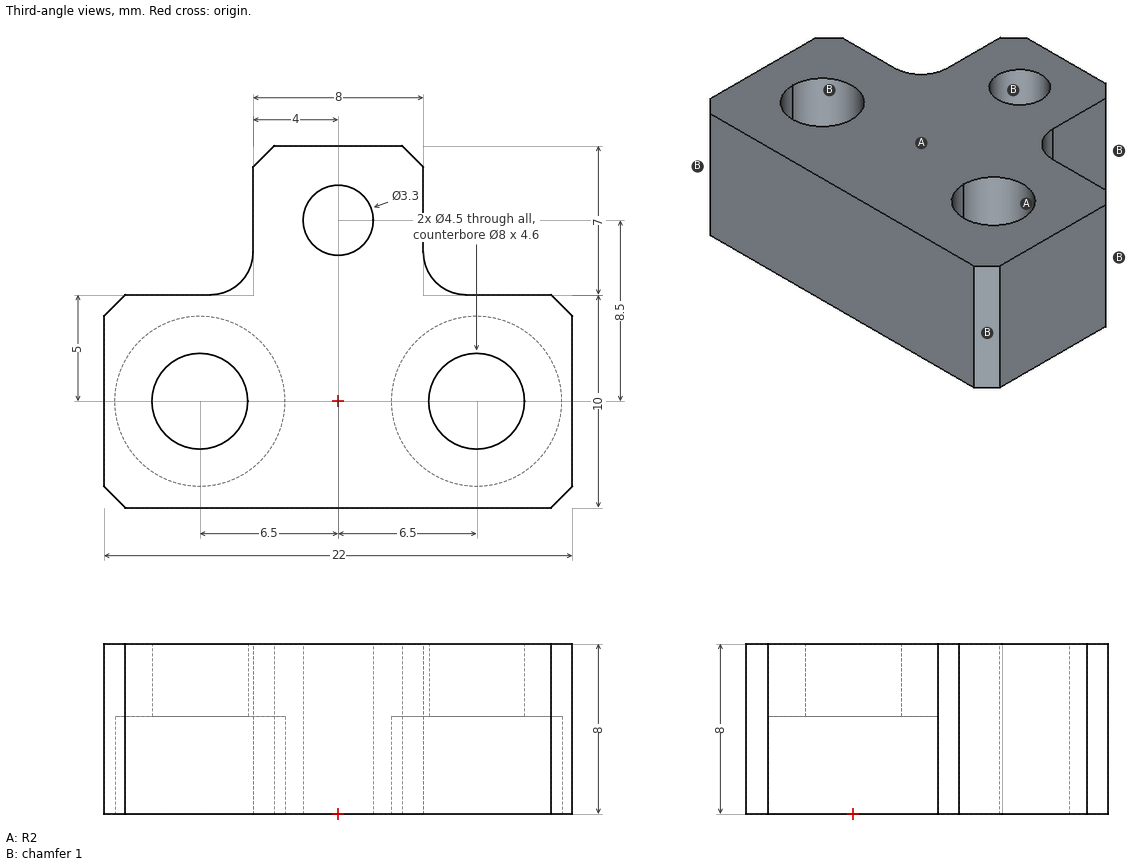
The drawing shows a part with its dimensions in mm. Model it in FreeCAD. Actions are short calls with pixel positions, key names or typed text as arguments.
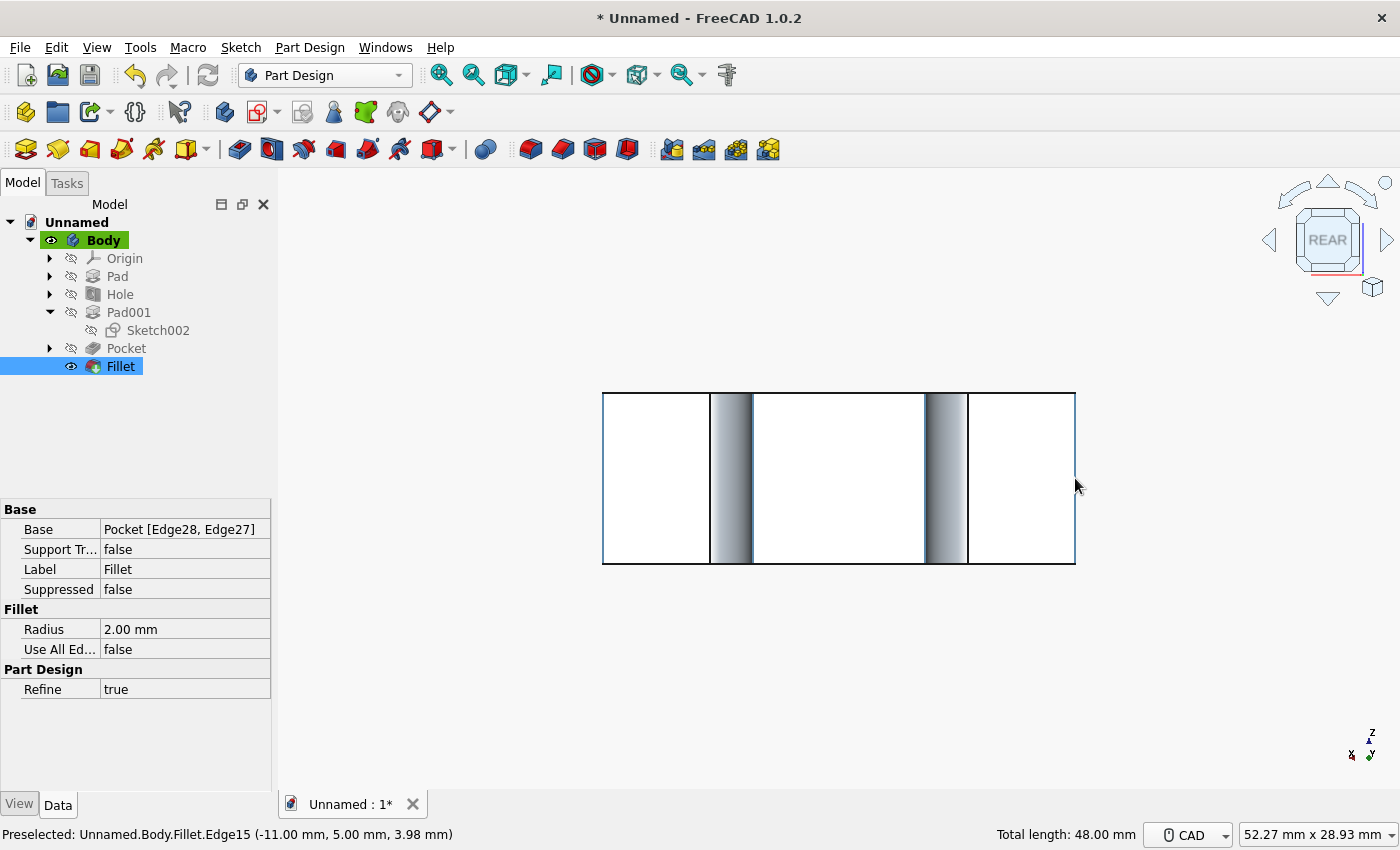
click(564, 150)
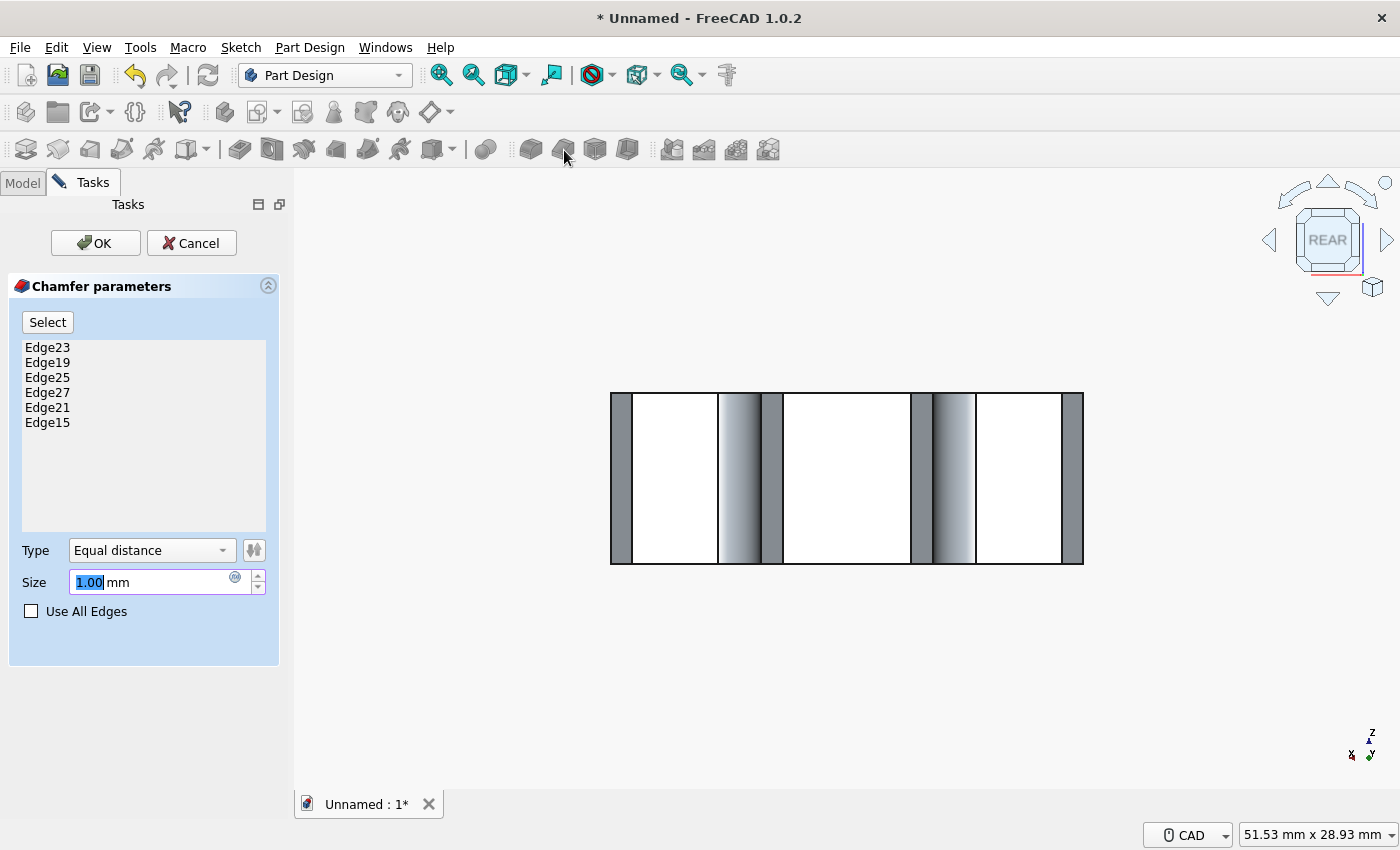
text(1)
key(Tab)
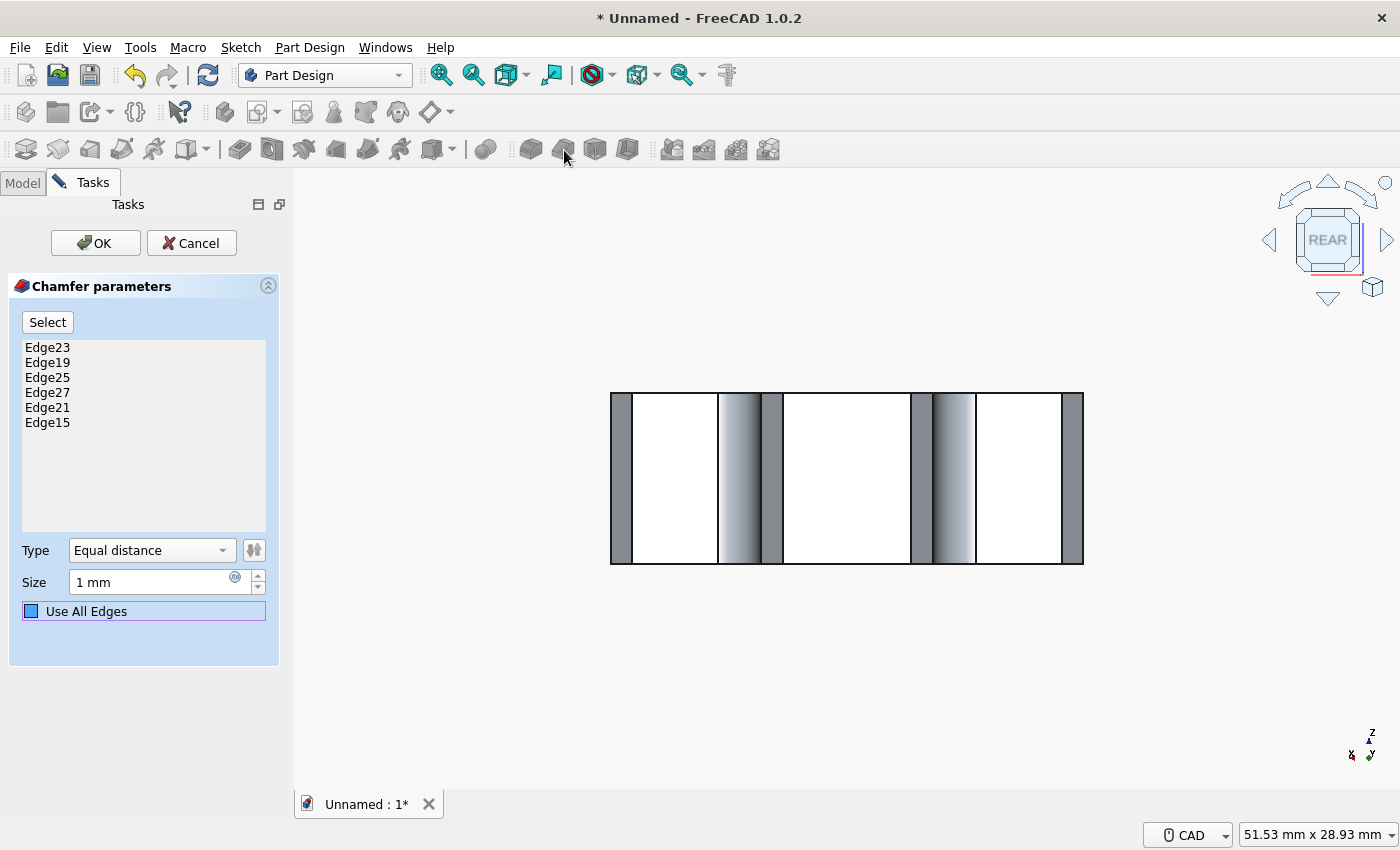
click(96, 243)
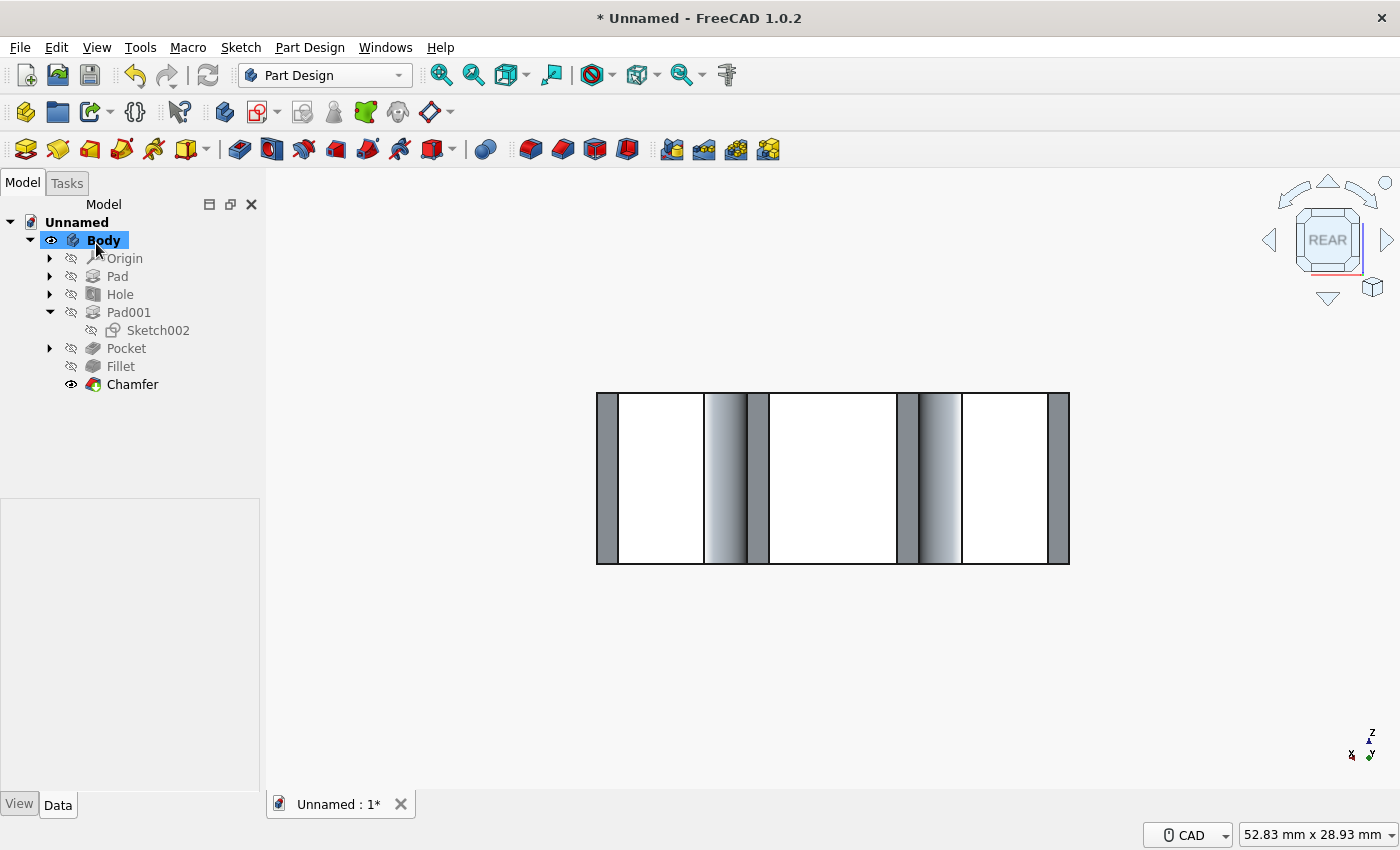
key(0)